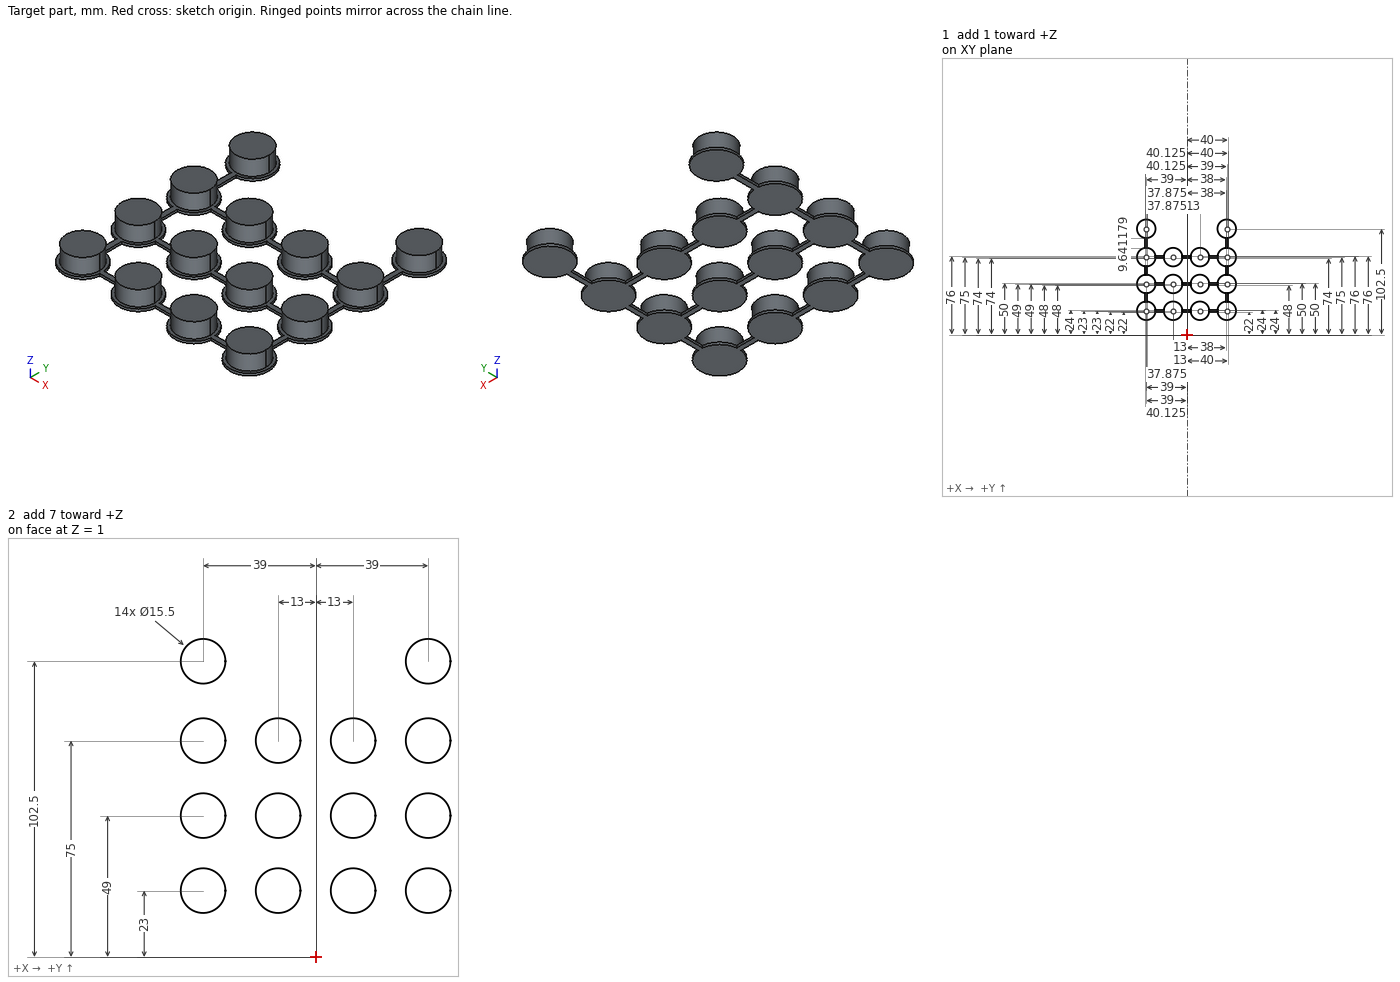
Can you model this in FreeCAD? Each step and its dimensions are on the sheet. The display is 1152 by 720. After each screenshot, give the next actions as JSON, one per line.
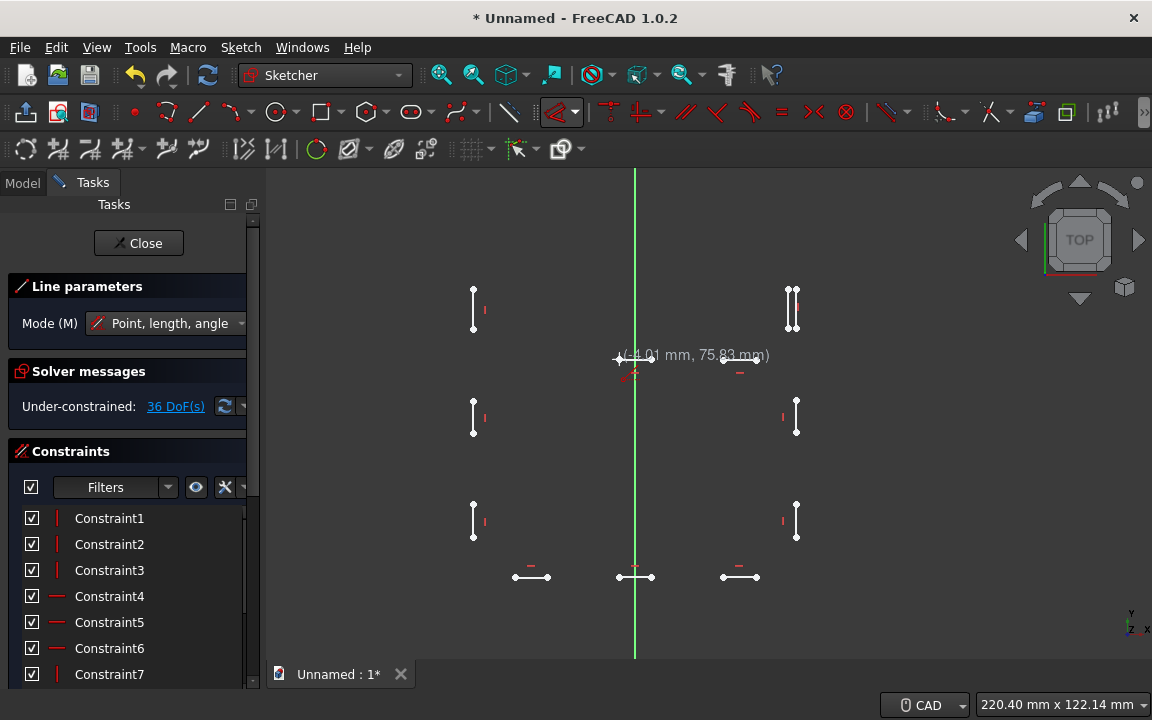
{"action": "left_click", "coordinate": [547, 359]}
{"action": "left_click", "coordinate": [514, 359]}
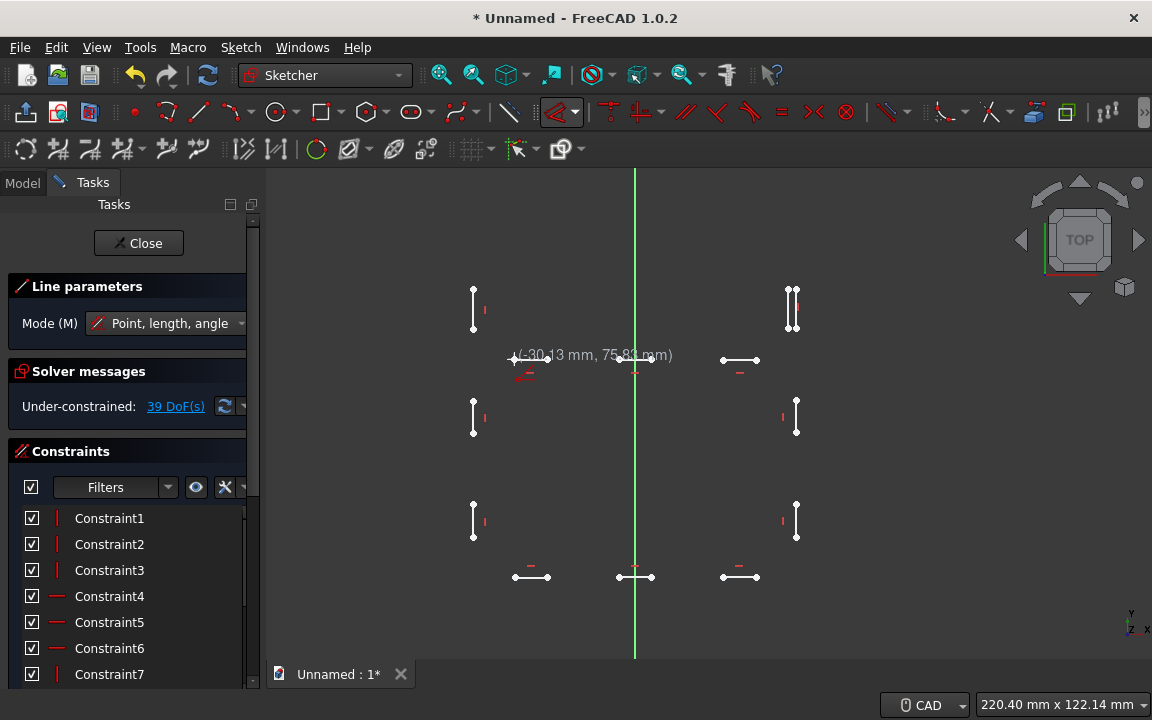
{"action": "scroll", "coordinate": [483, 327], "scroll_direction": "up", "scroll_amount": 3}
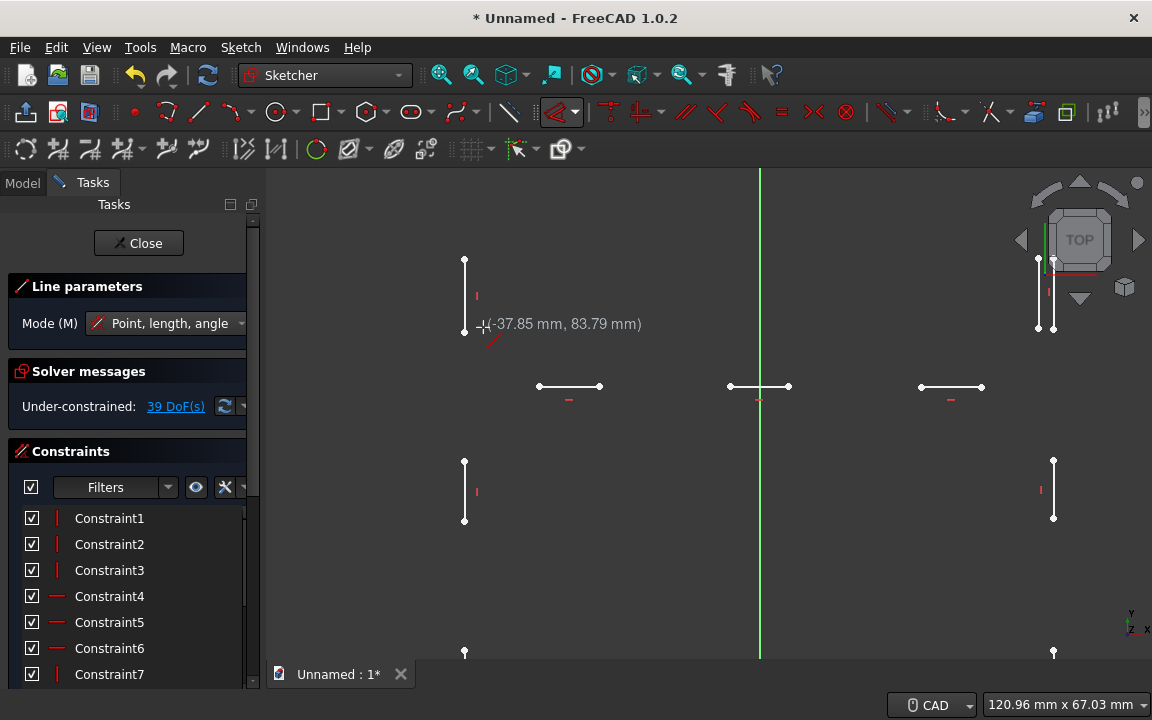
{"action": "left_click", "coordinate": [483, 328]}
{"action": "left_click", "coordinate": [483, 257]}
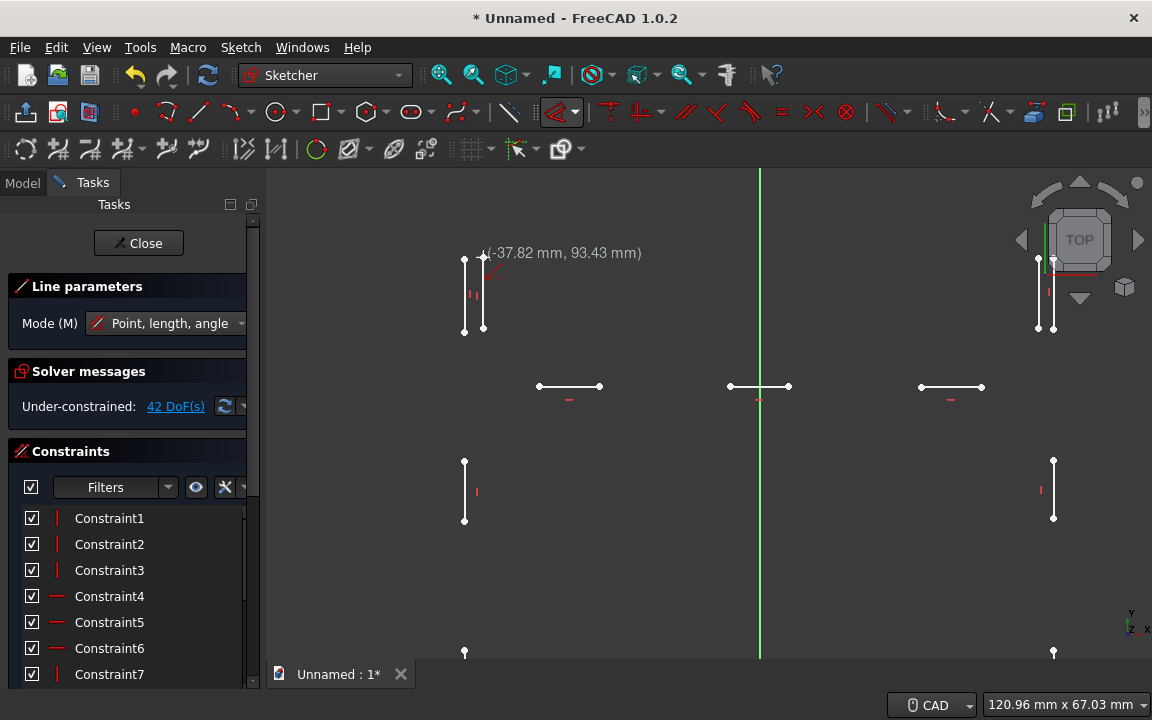
{"action": "left_click", "coordinate": [232, 112]}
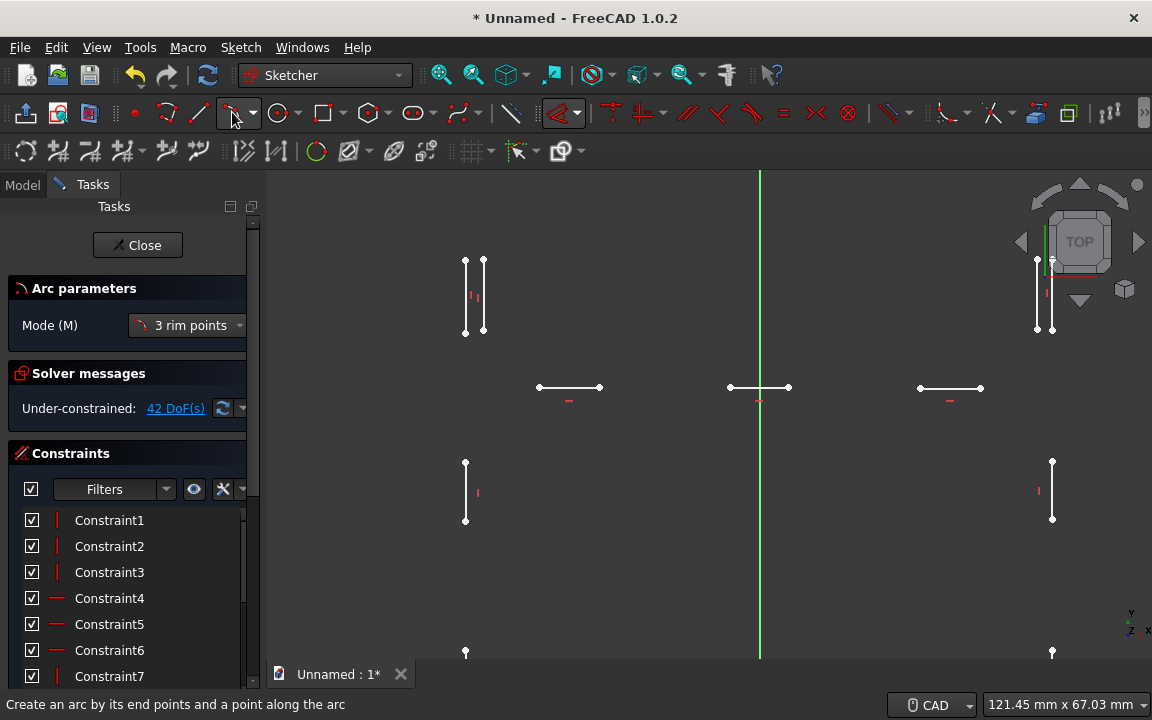
{"action": "left_click", "coordinate": [466, 333]}
{"action": "left_click", "coordinate": [466, 462]}
{"action": "left_click", "coordinate": [410, 394]}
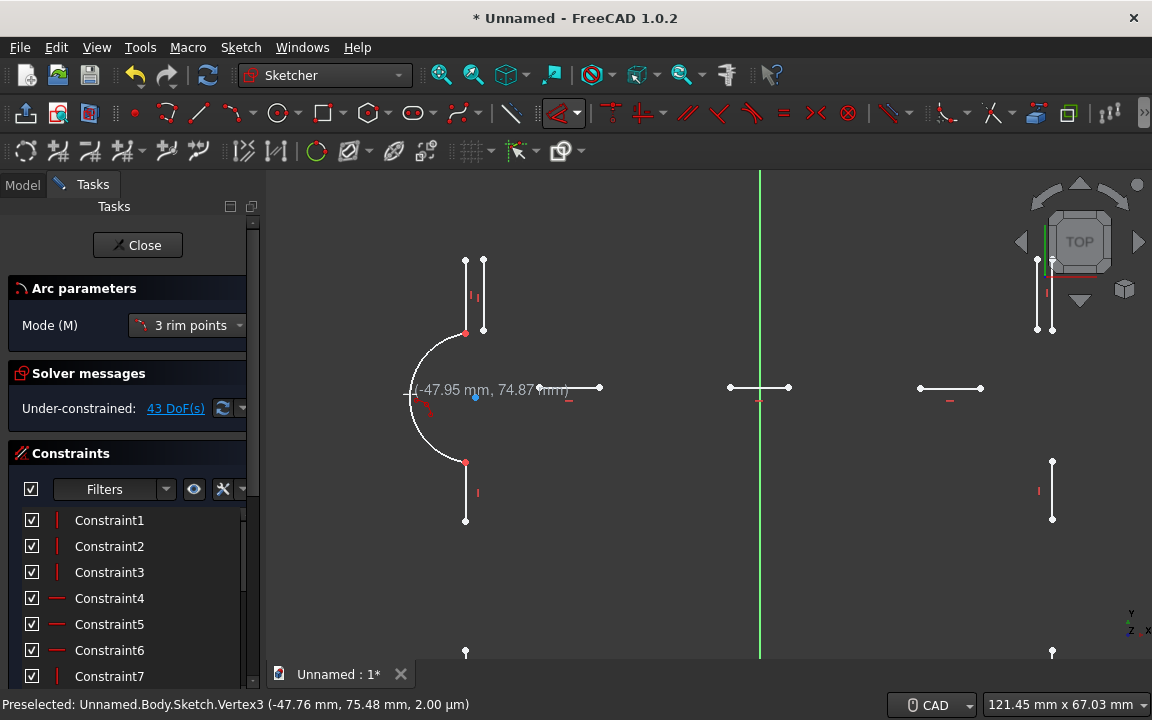
{"action": "left_click", "coordinate": [466, 522]}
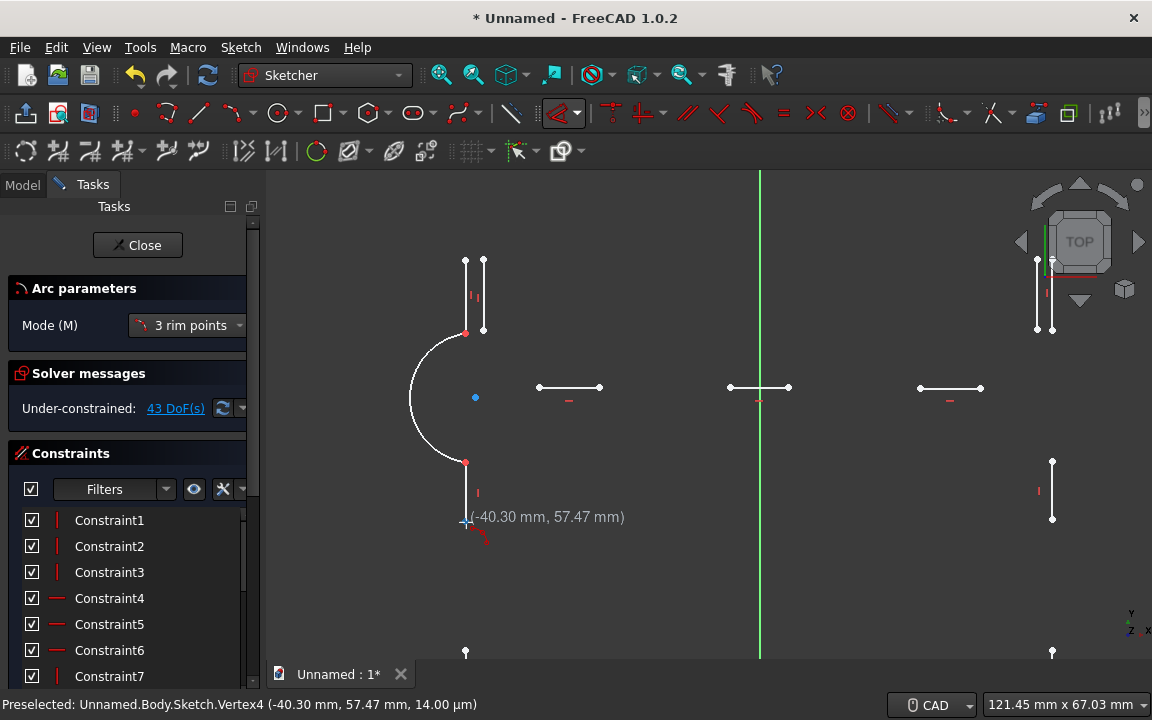
{"action": "scroll", "coordinate": [571, 345], "scroll_direction": "down", "scroll_amount": 5}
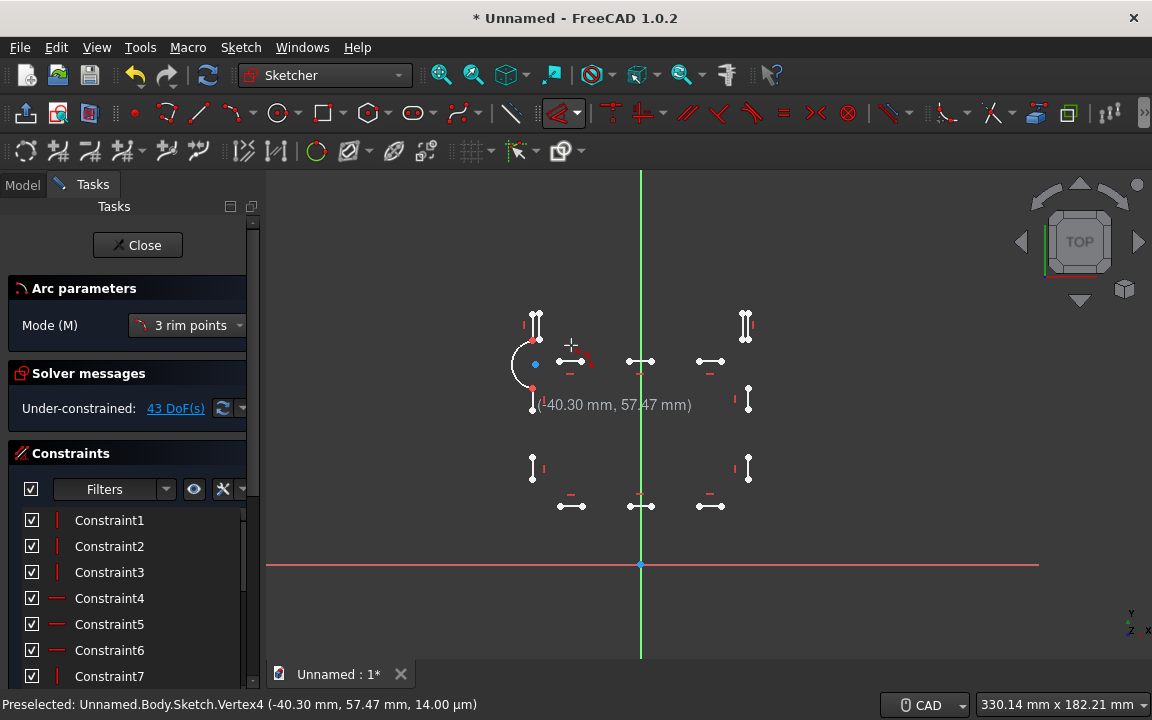
{"action": "scroll", "coordinate": [533, 457], "scroll_direction": "up", "scroll_amount": 2}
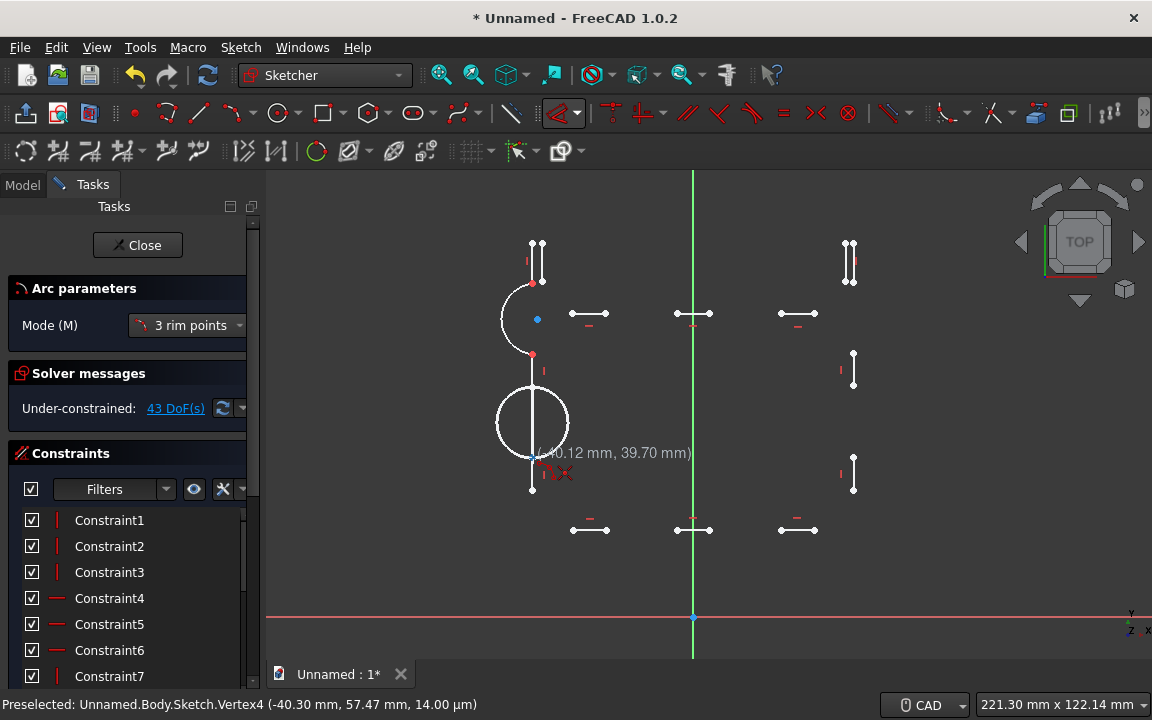
{"action": "left_click", "coordinate": [532, 458]}
{"action": "left_click", "coordinate": [501, 421]}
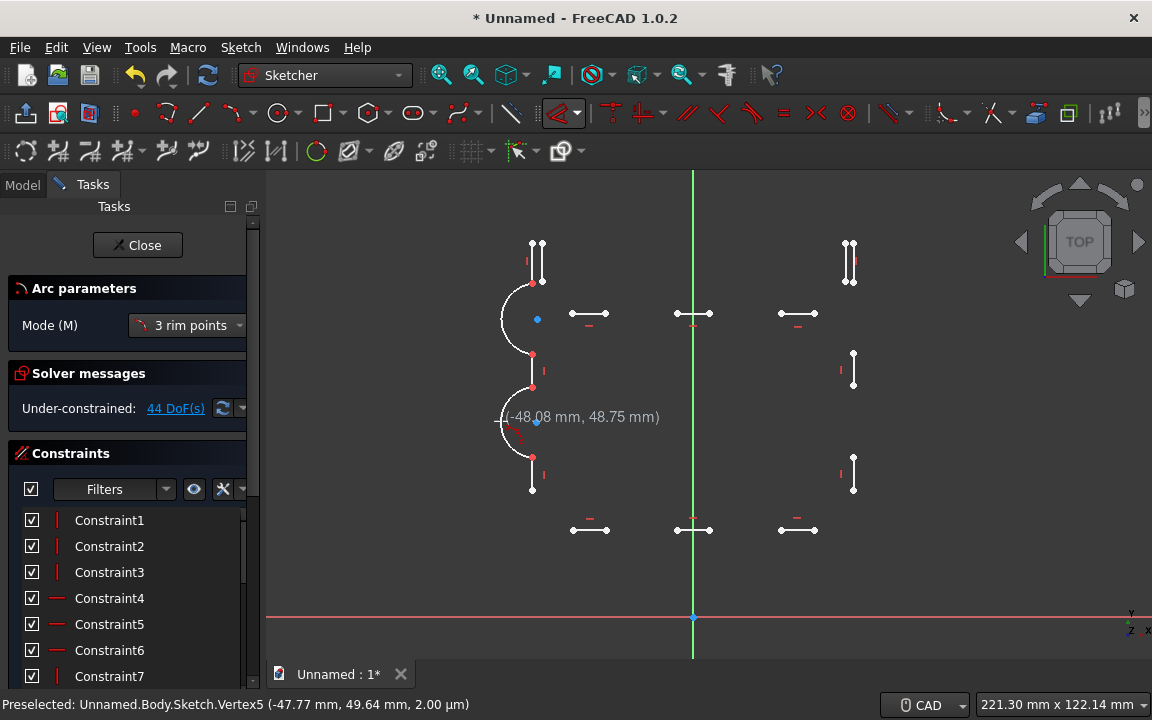
{"action": "left_click", "coordinate": [532, 491]}
{"action": "left_click", "coordinate": [574, 530]}
{"action": "left_click", "coordinate": [512, 551]}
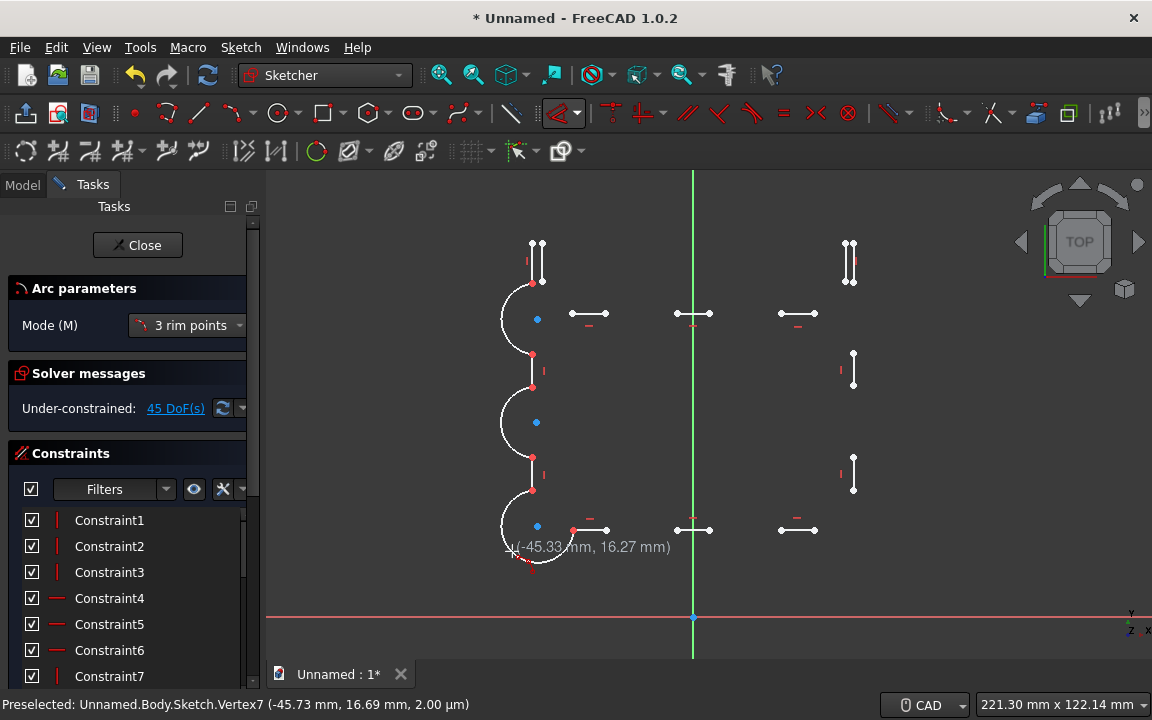
{"action": "left_click", "coordinate": [607, 530]}
{"action": "left_click", "coordinate": [678, 530]}
{"action": "left_click", "coordinate": [641, 561]}